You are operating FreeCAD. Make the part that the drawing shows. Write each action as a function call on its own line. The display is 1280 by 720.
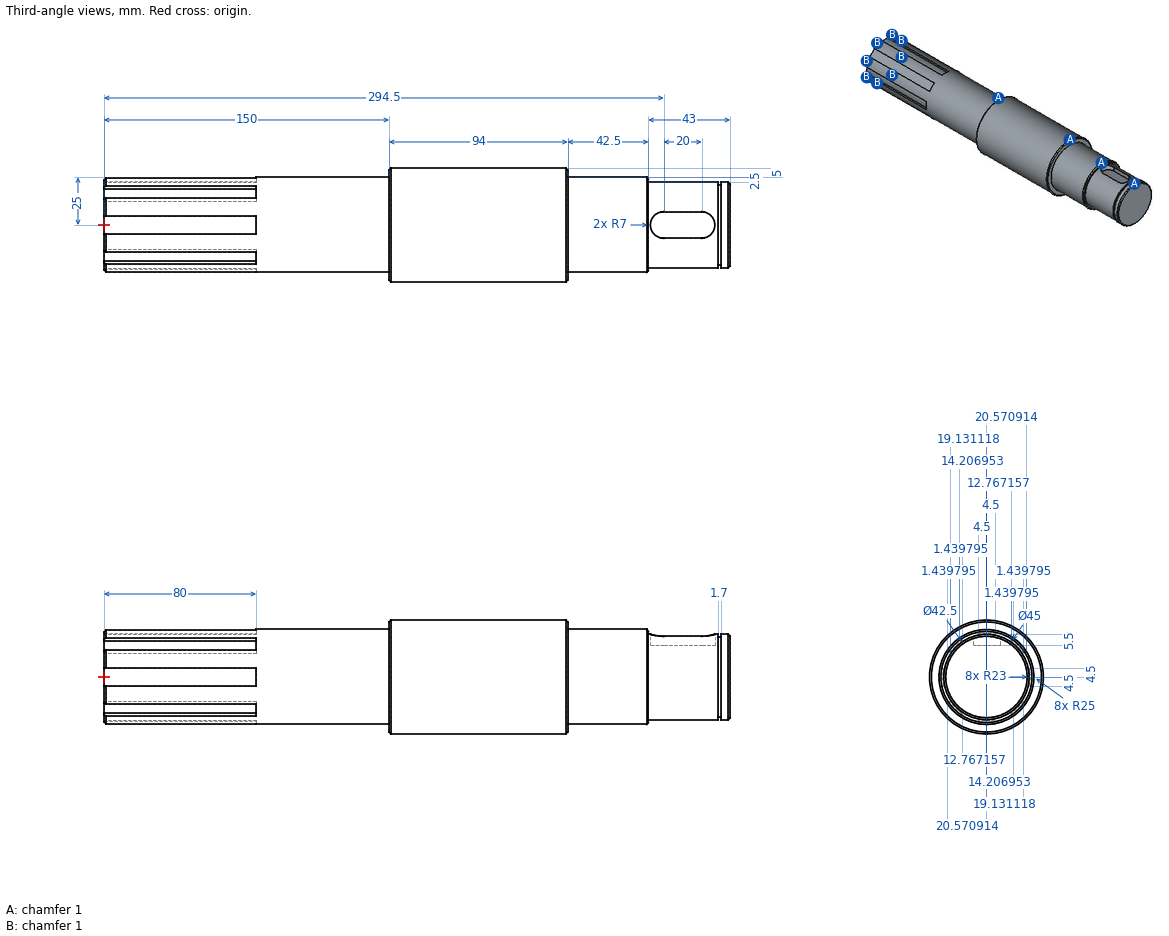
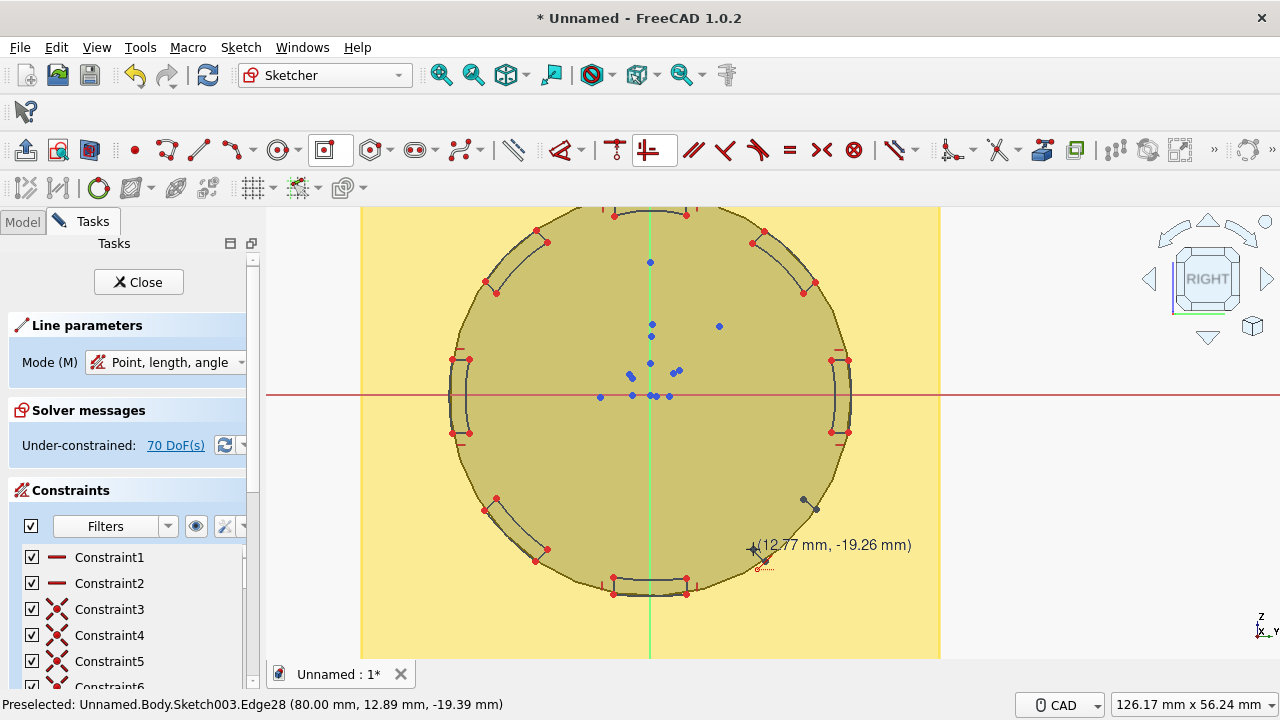
click(232, 150)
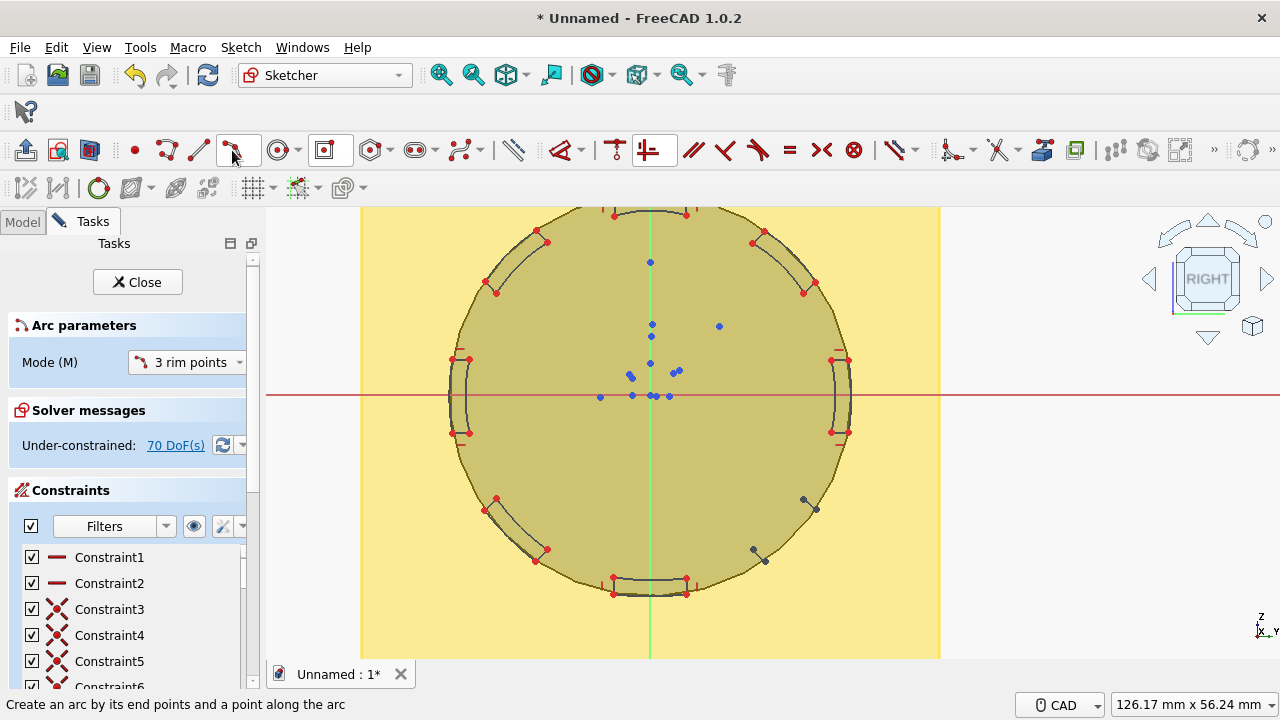
scroll(816, 509, up, 4)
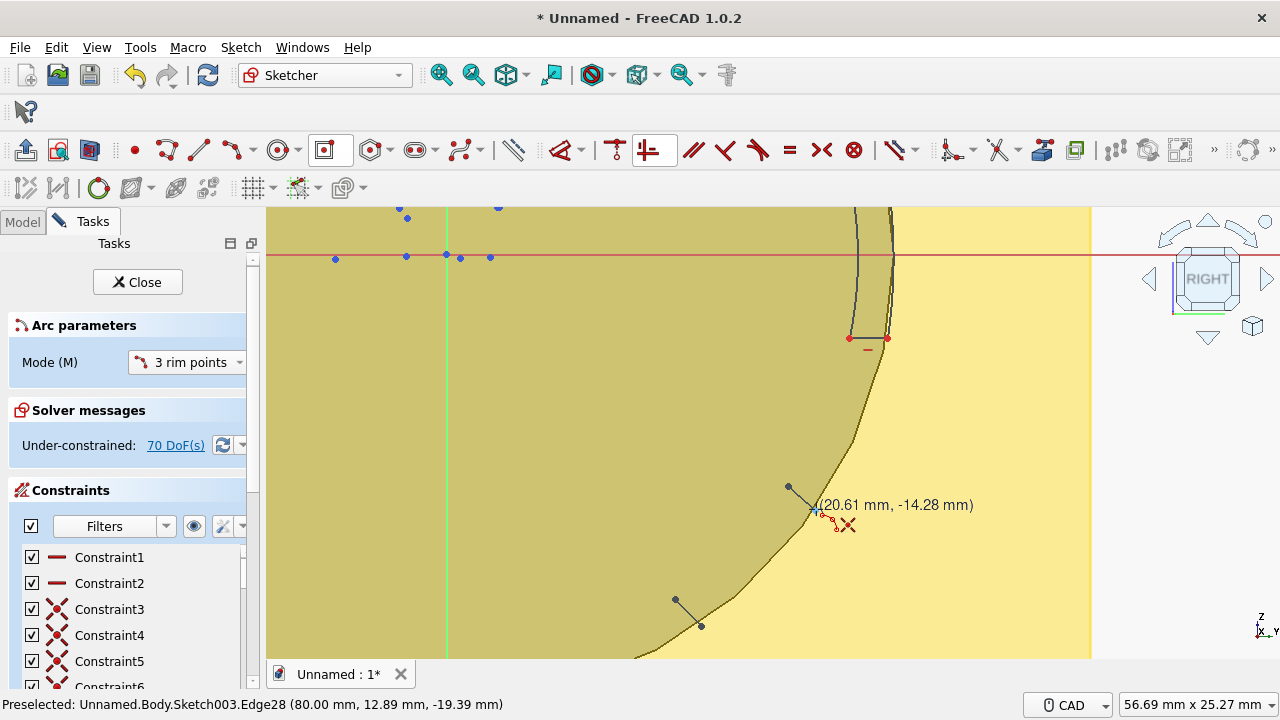
click(815, 510)
click(702, 626)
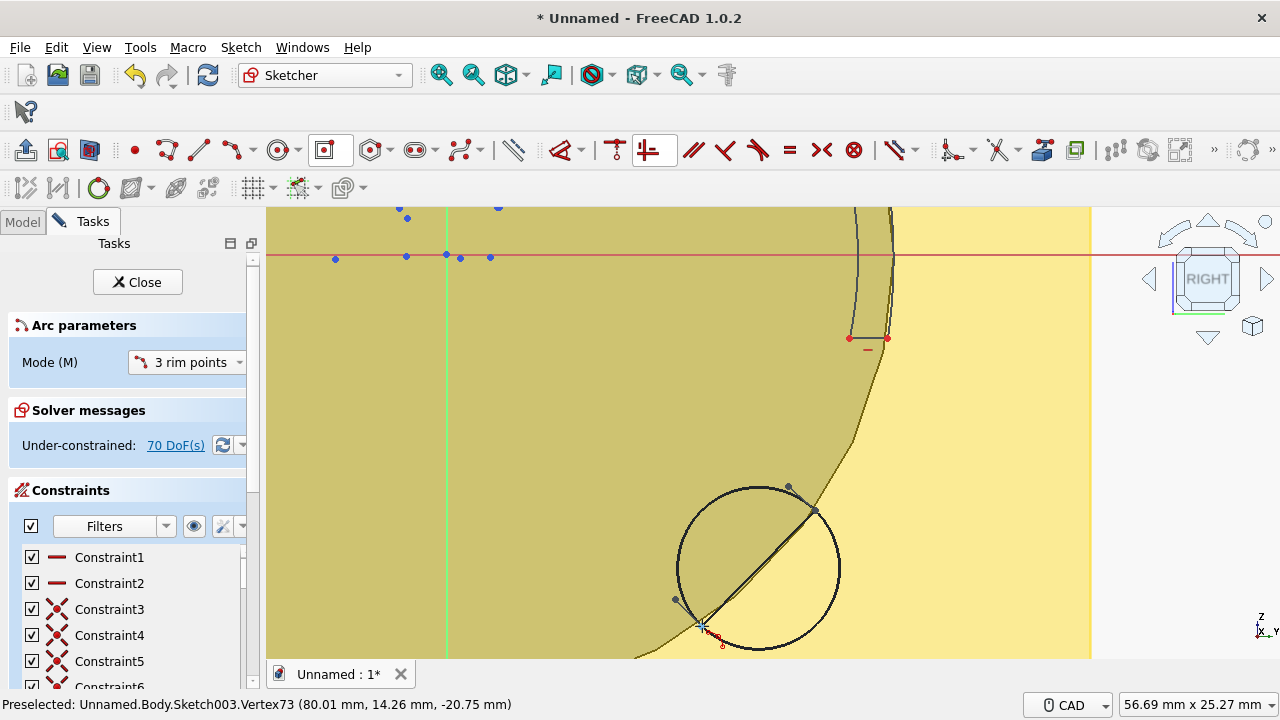
scroll(763, 571, up, 4)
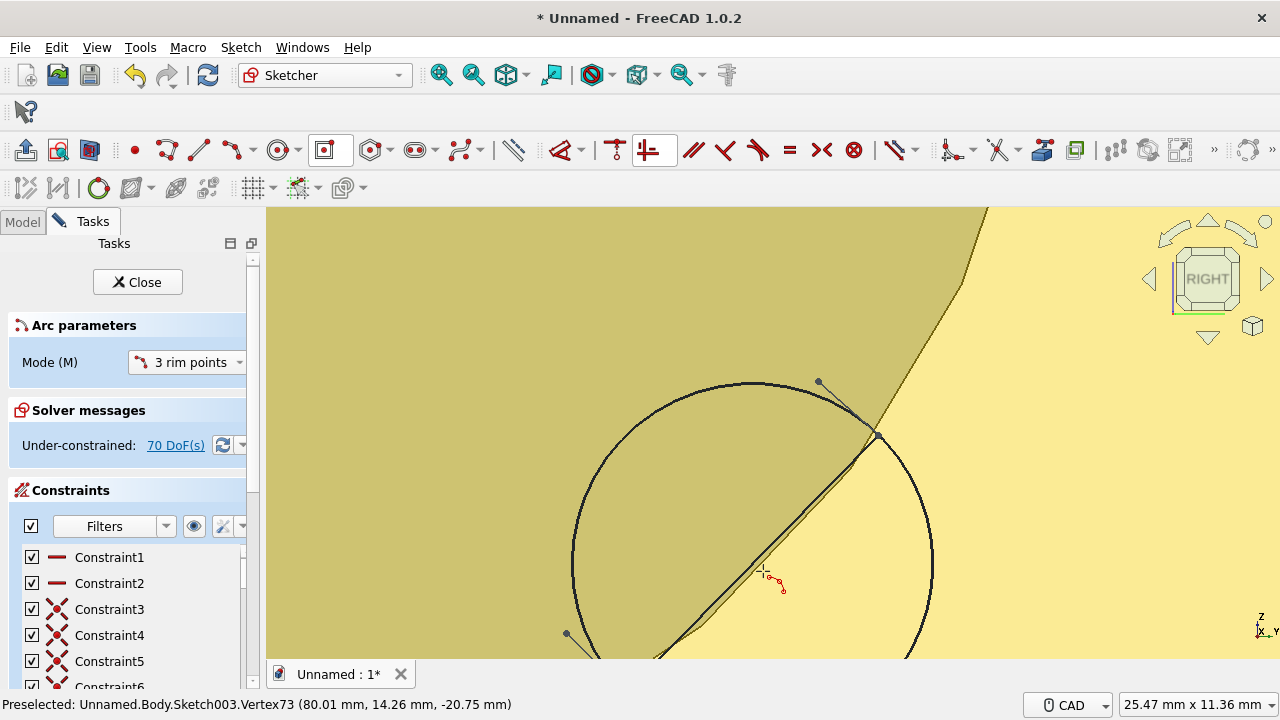
click(762, 570)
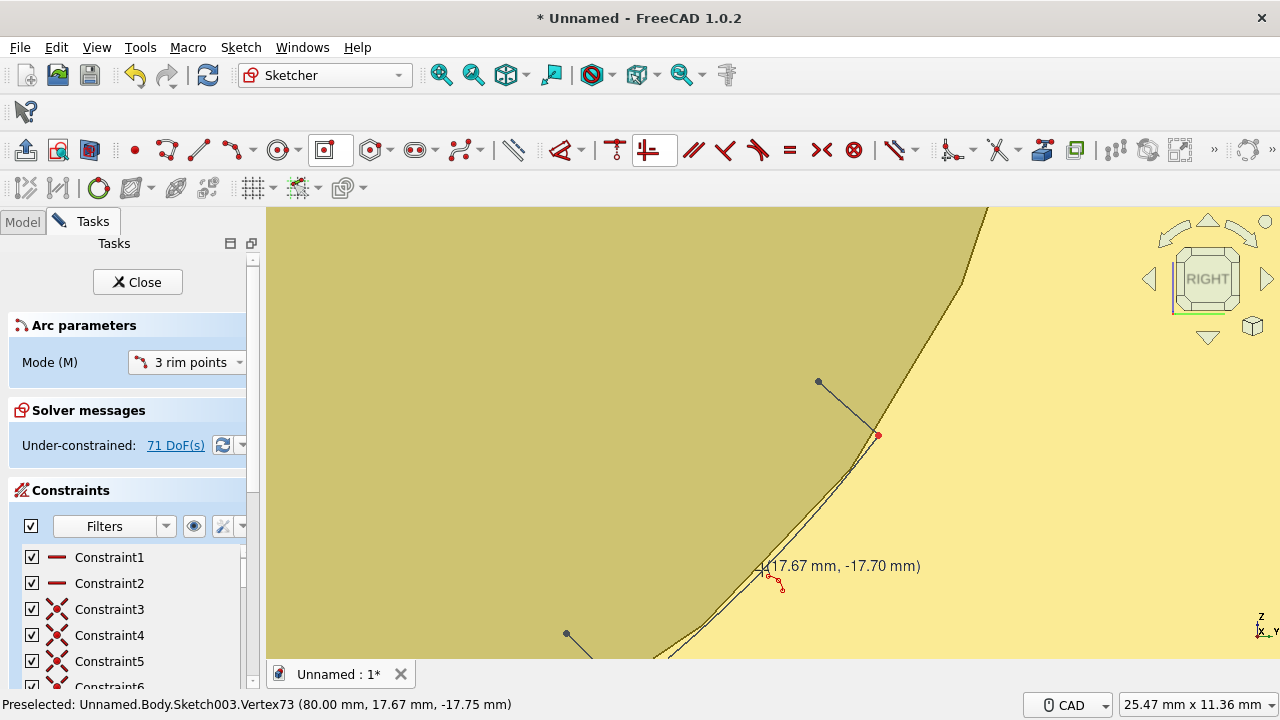
click(567, 633)
click(818, 382)
click(706, 514)
key(Escape)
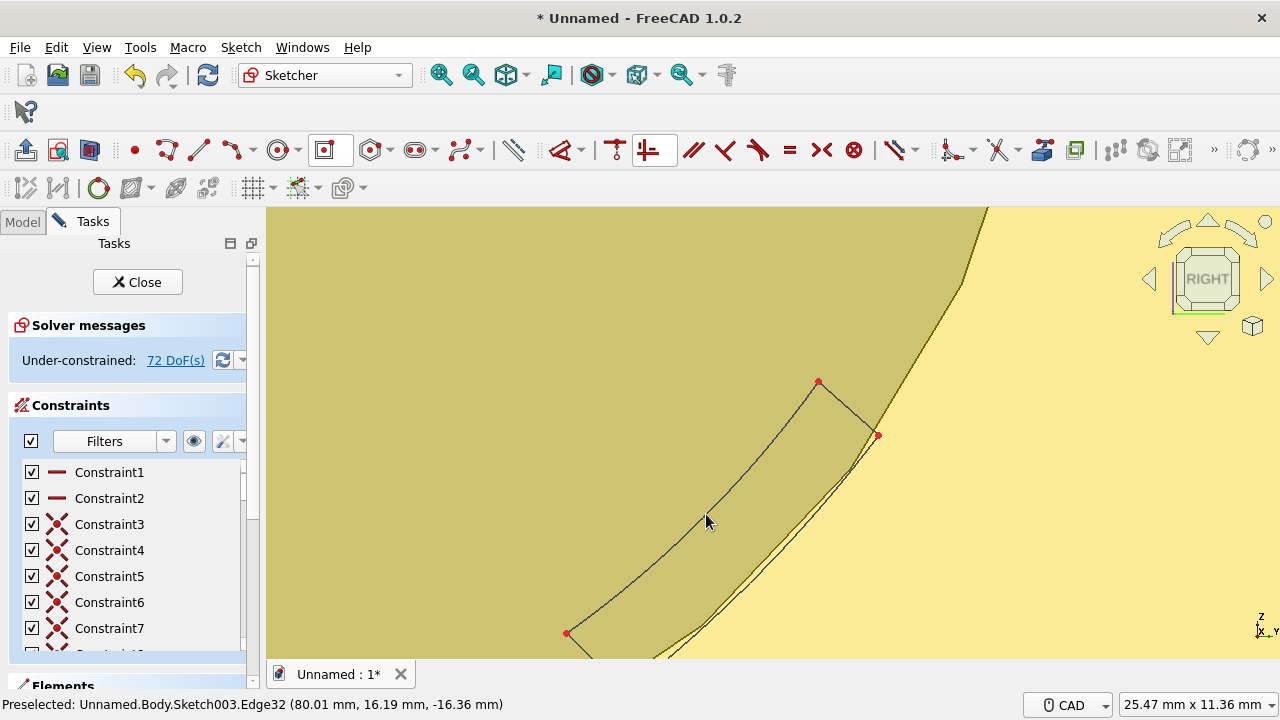
scroll(806, 522, down, 10)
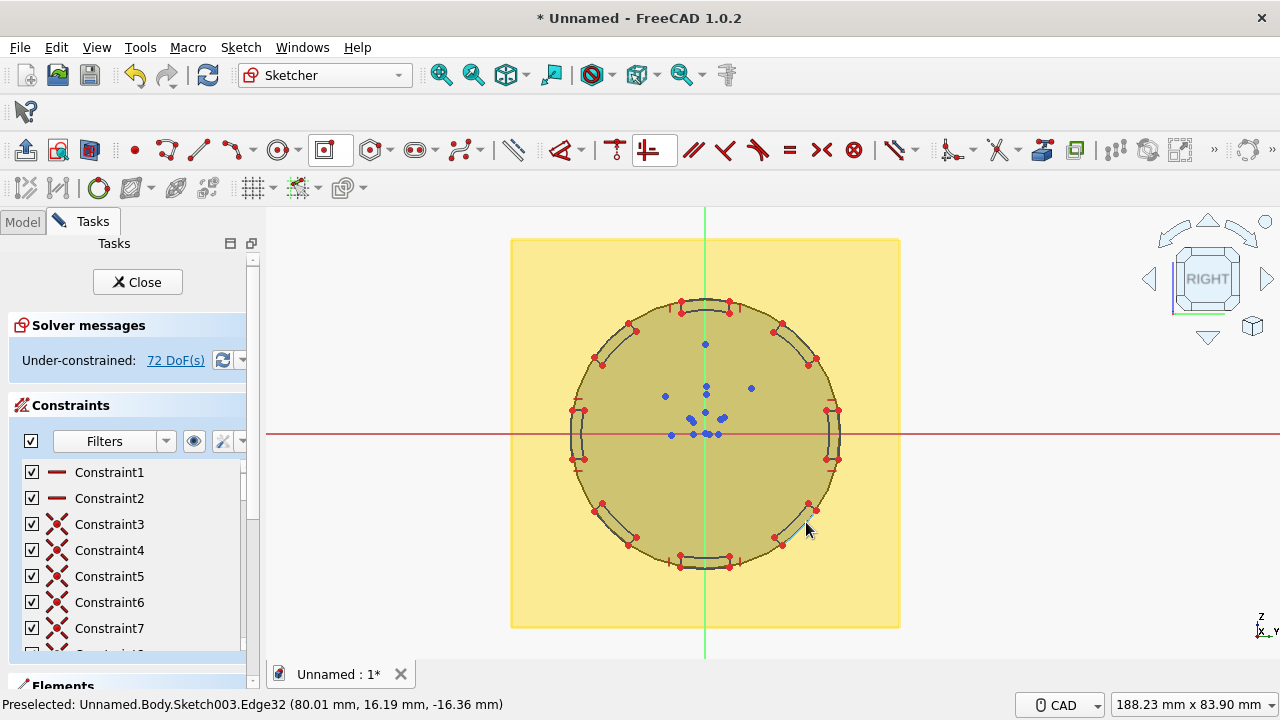
scroll(829, 445, up, 2)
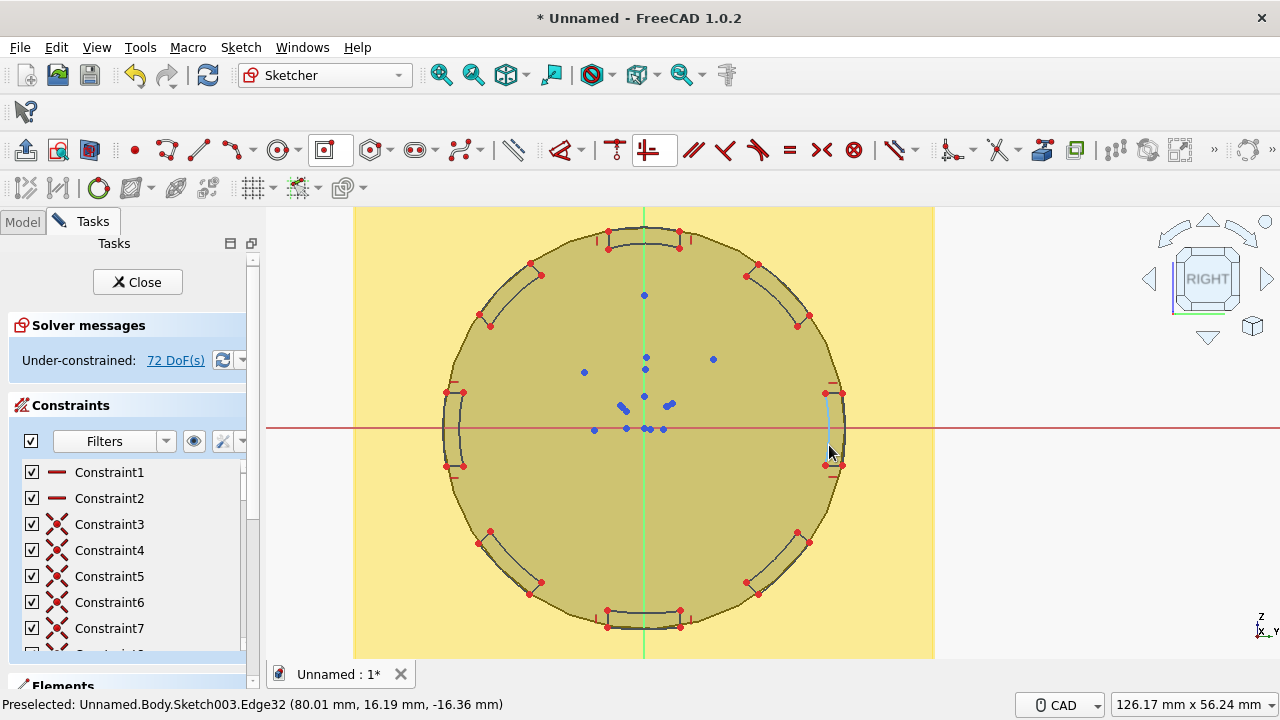
click(828, 444)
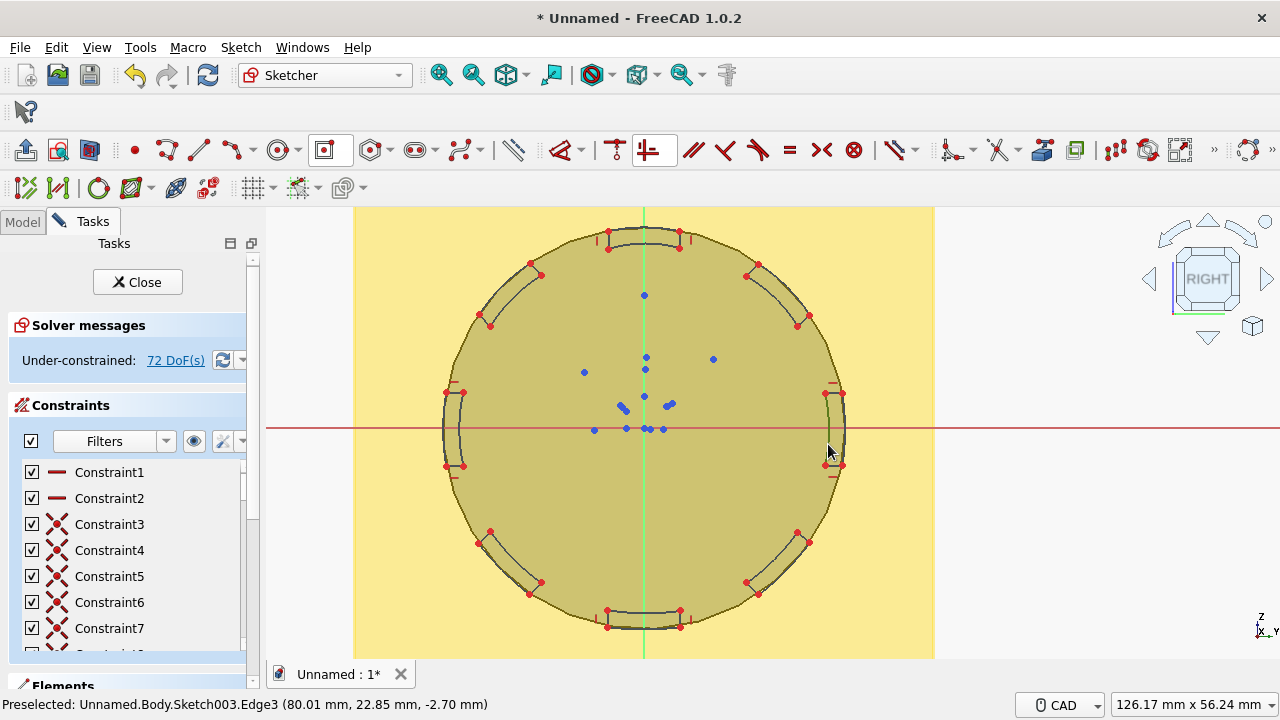
click(845, 444)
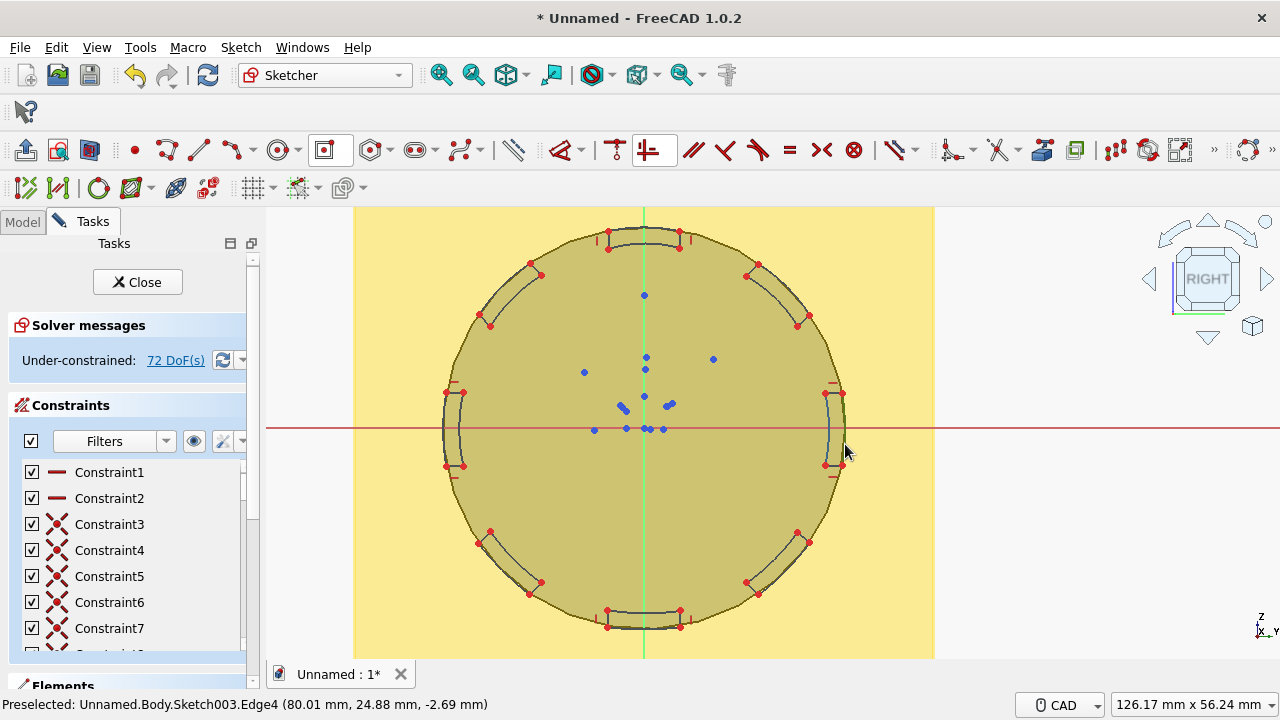
click(616, 150)